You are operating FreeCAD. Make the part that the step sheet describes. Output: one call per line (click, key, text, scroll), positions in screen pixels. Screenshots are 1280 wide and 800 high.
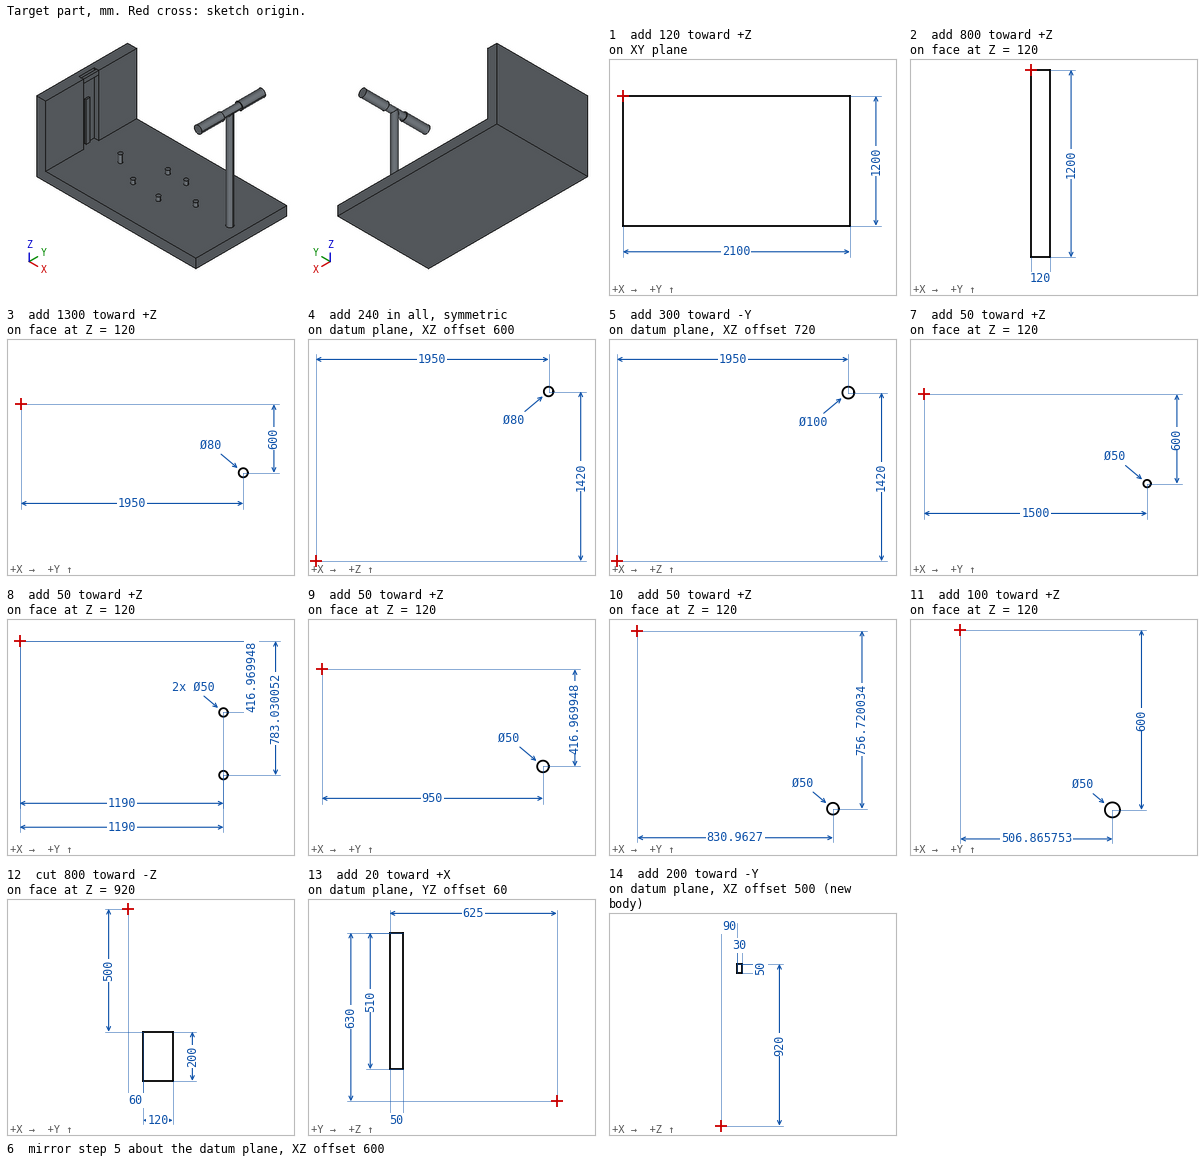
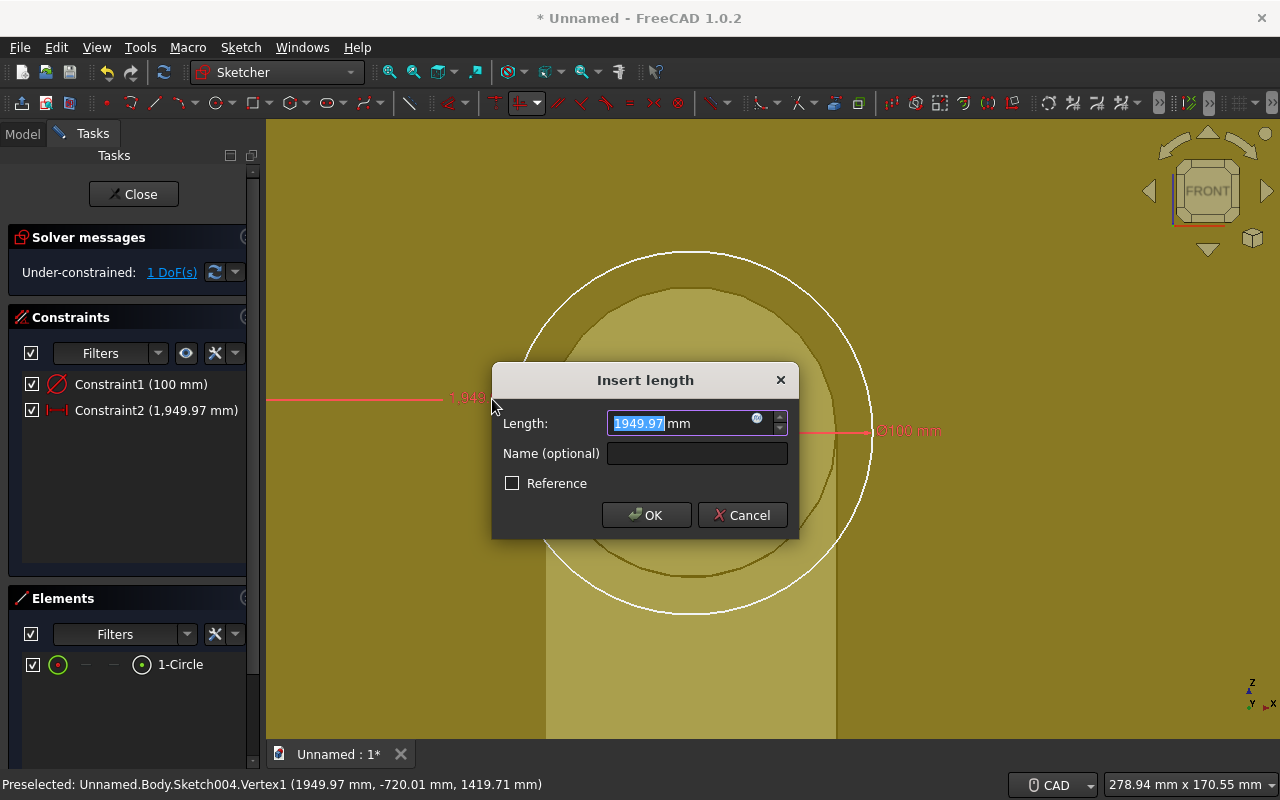
text(1950)
key(Return)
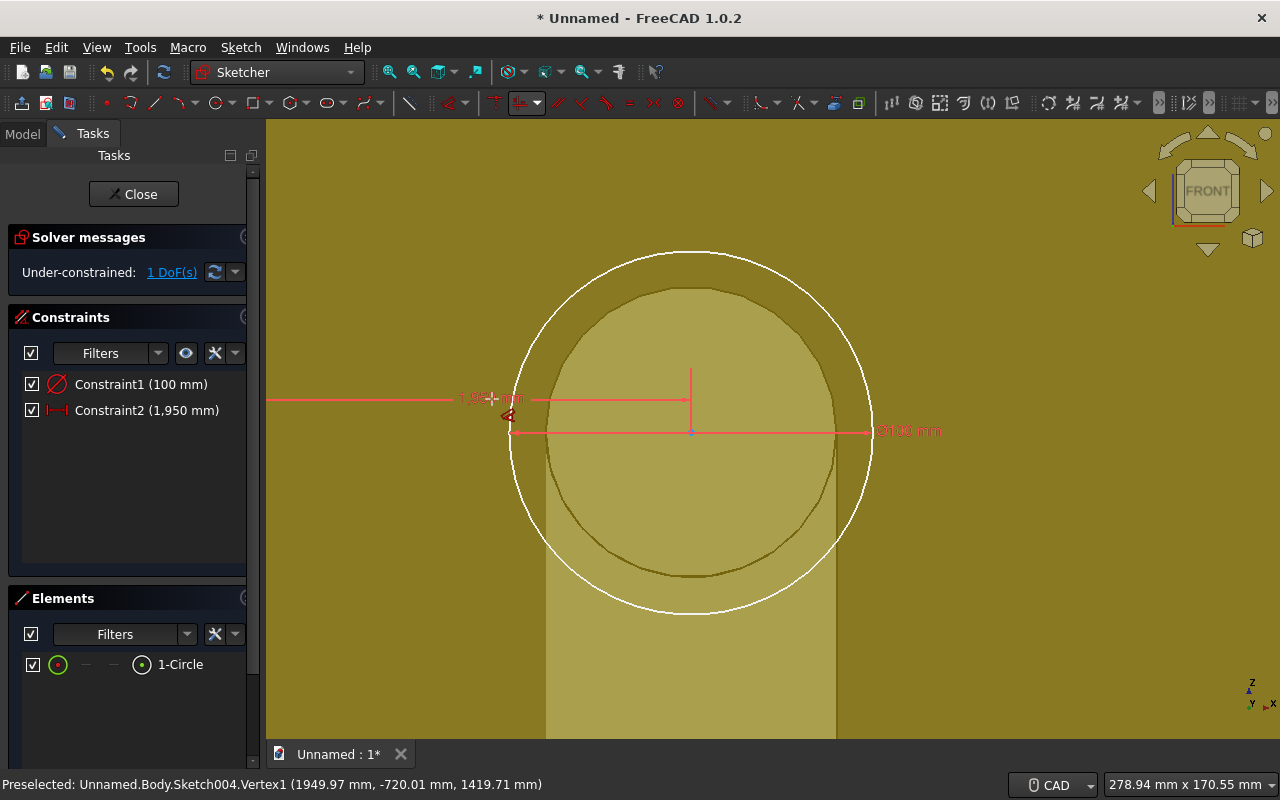
click(691, 433)
click(725, 572)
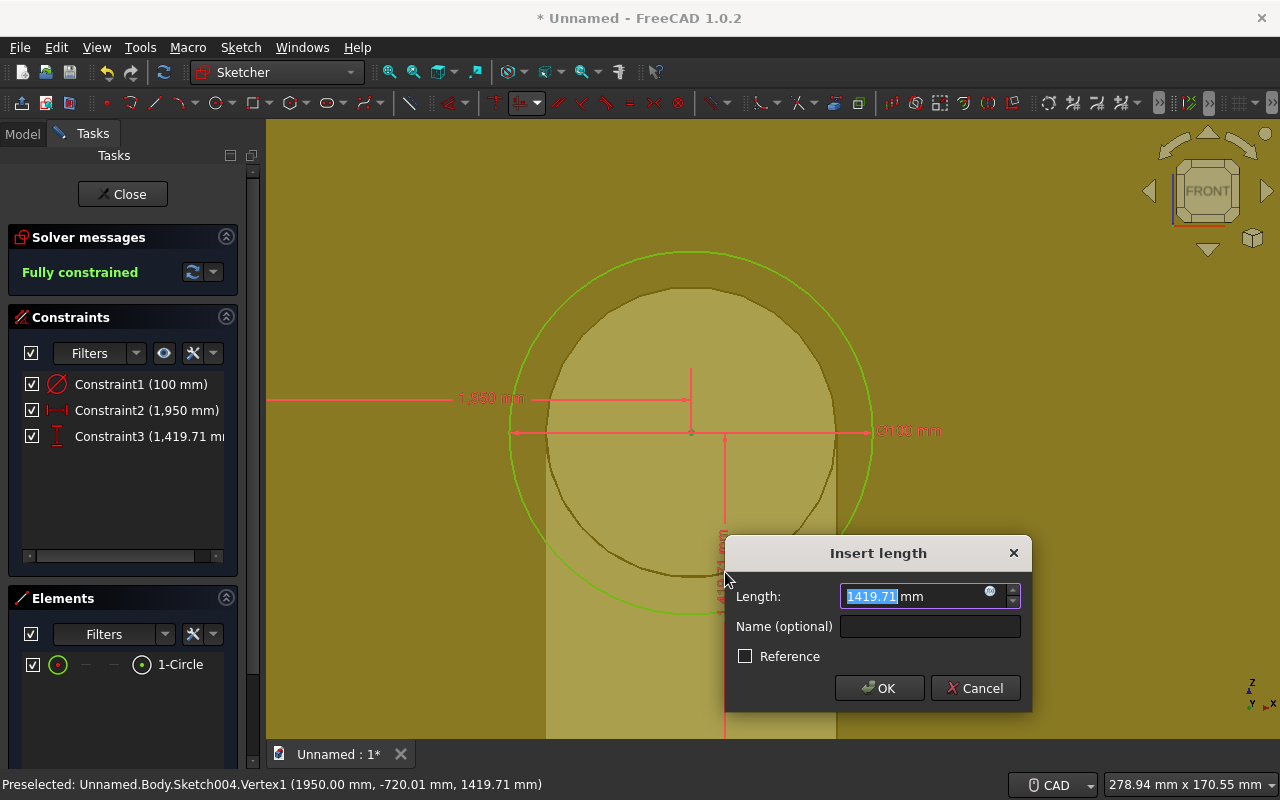
text(1420)
key(Return)
key(Escape)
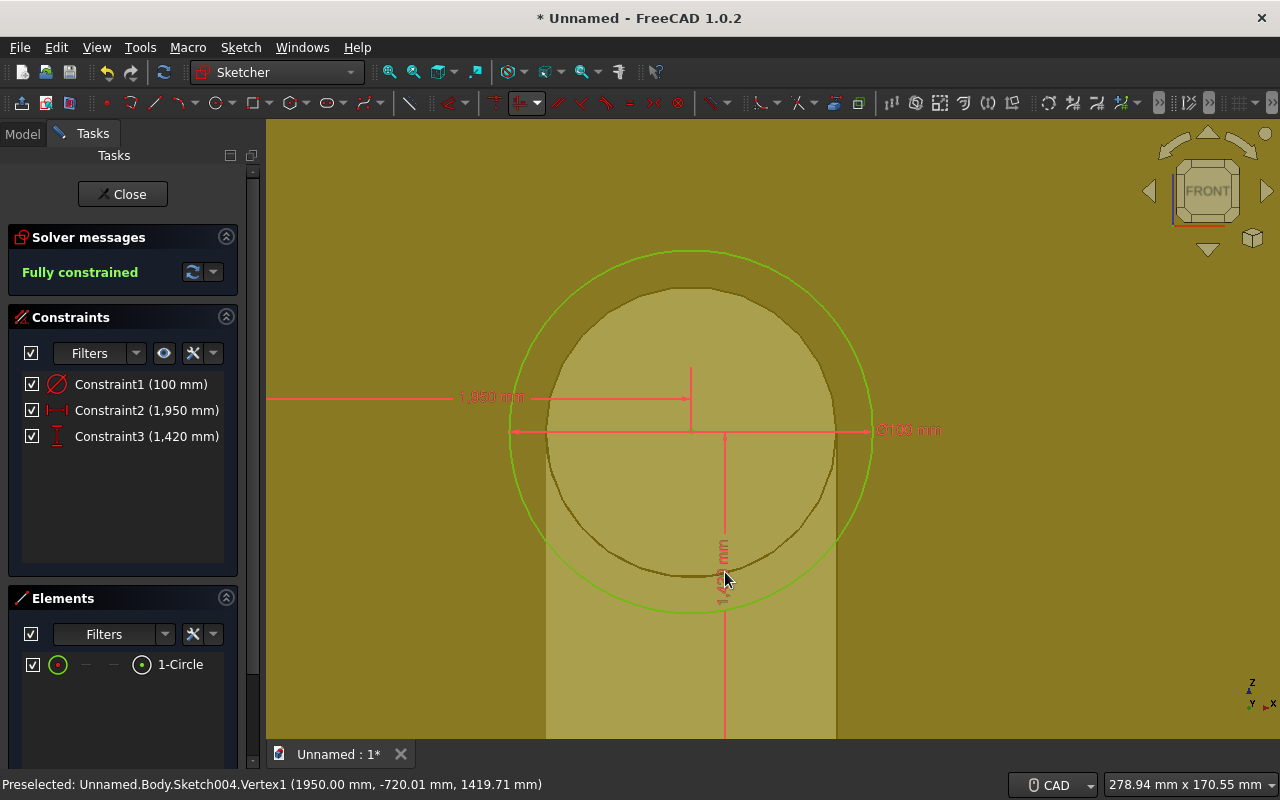
click(123, 194)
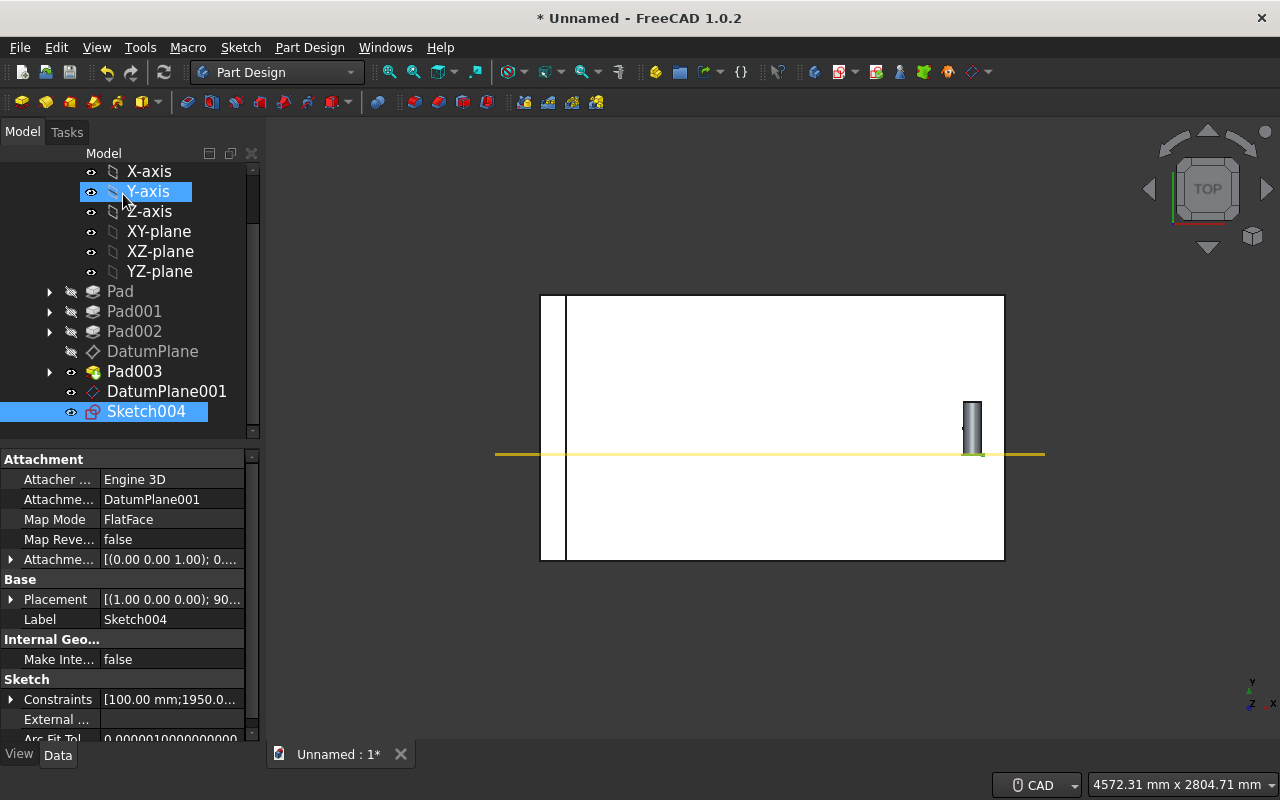
click(22, 102)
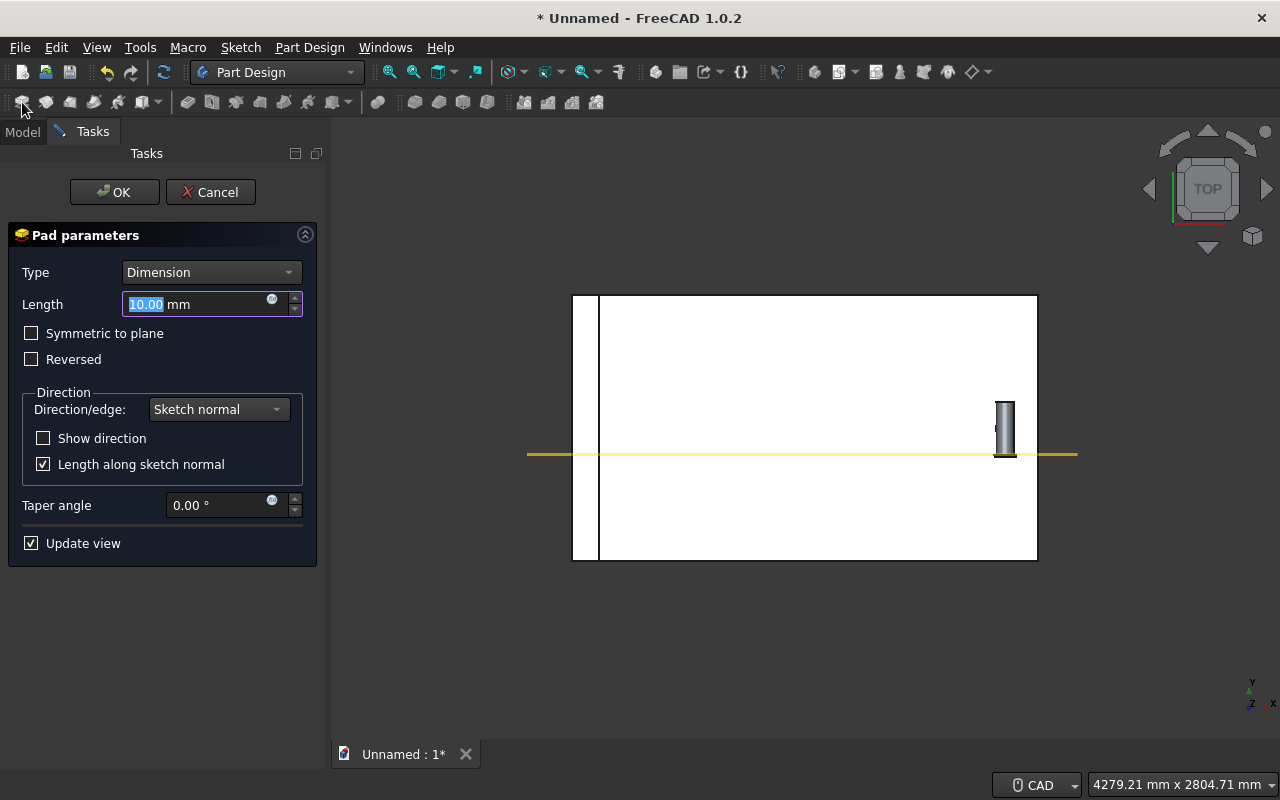
text(300)
key(Tab)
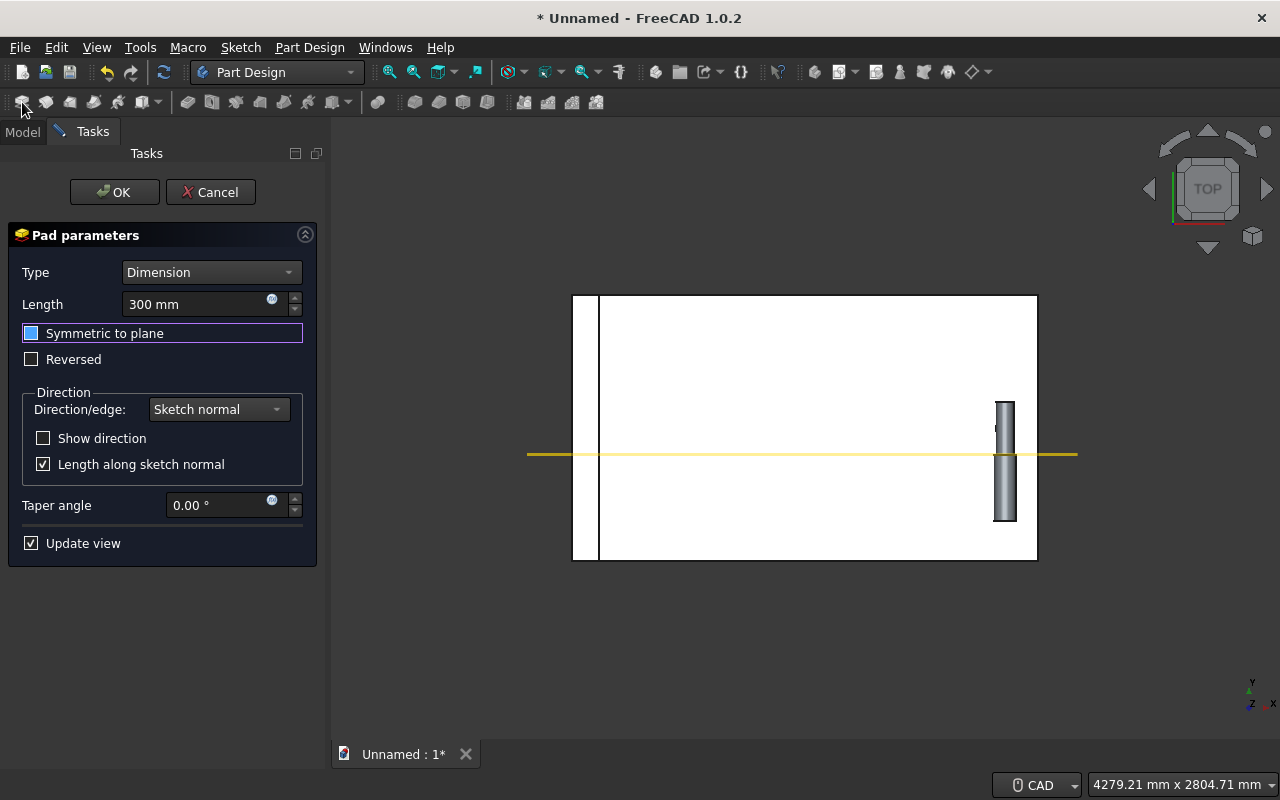
click(115, 192)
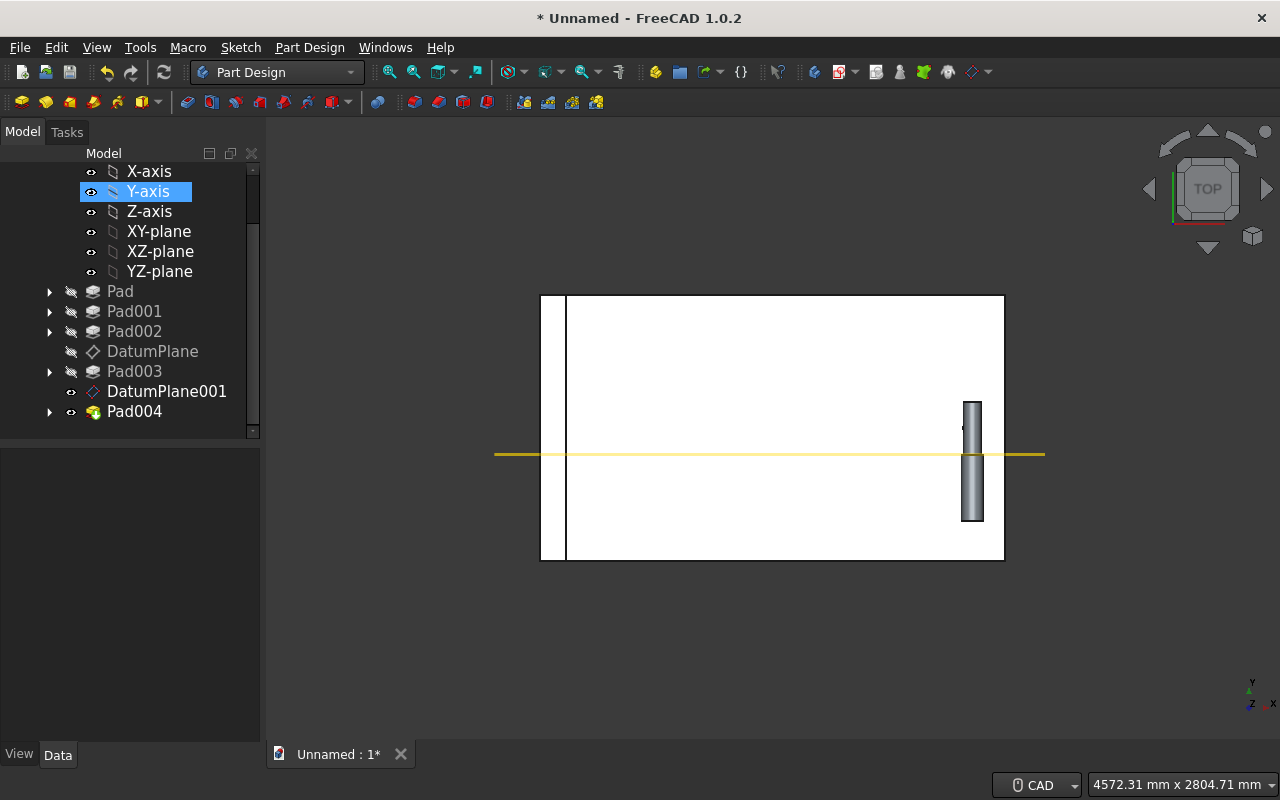
click(116, 392)
key(space)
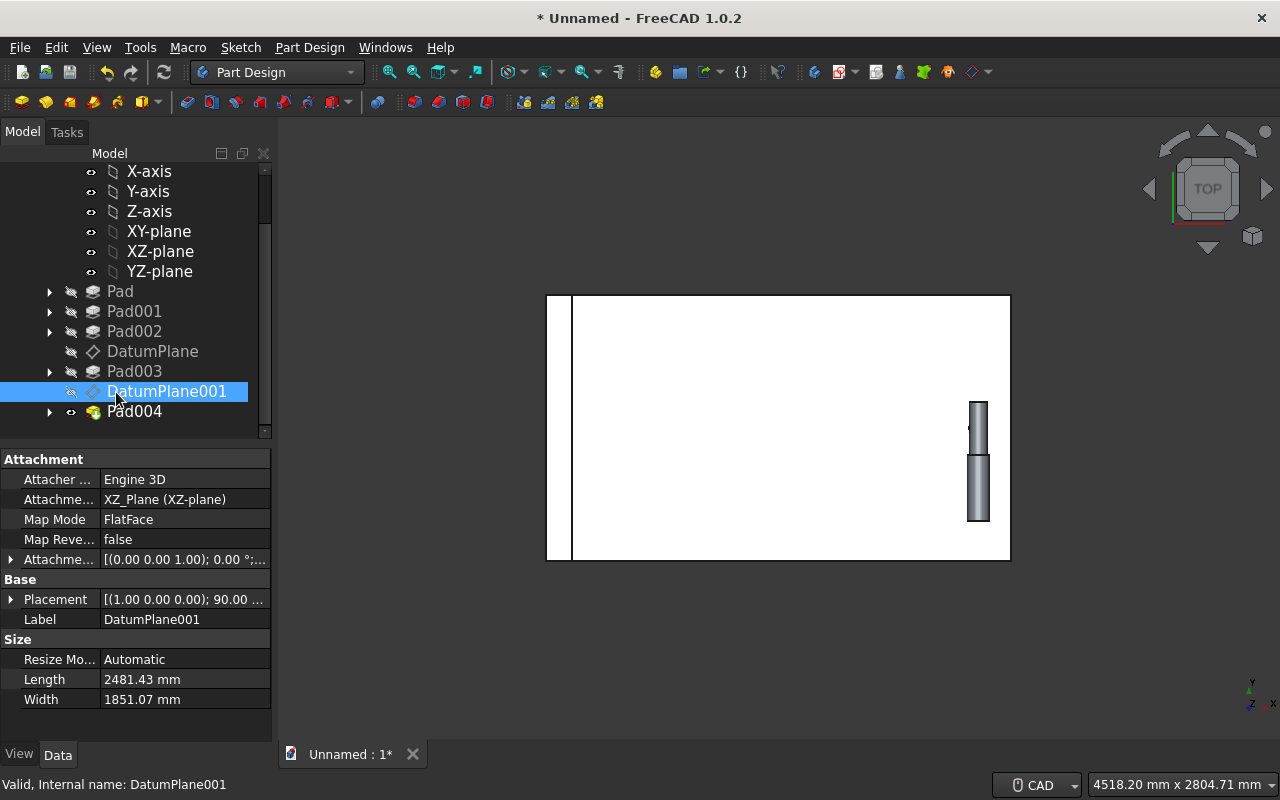
scroll(160, 287, down, 3)